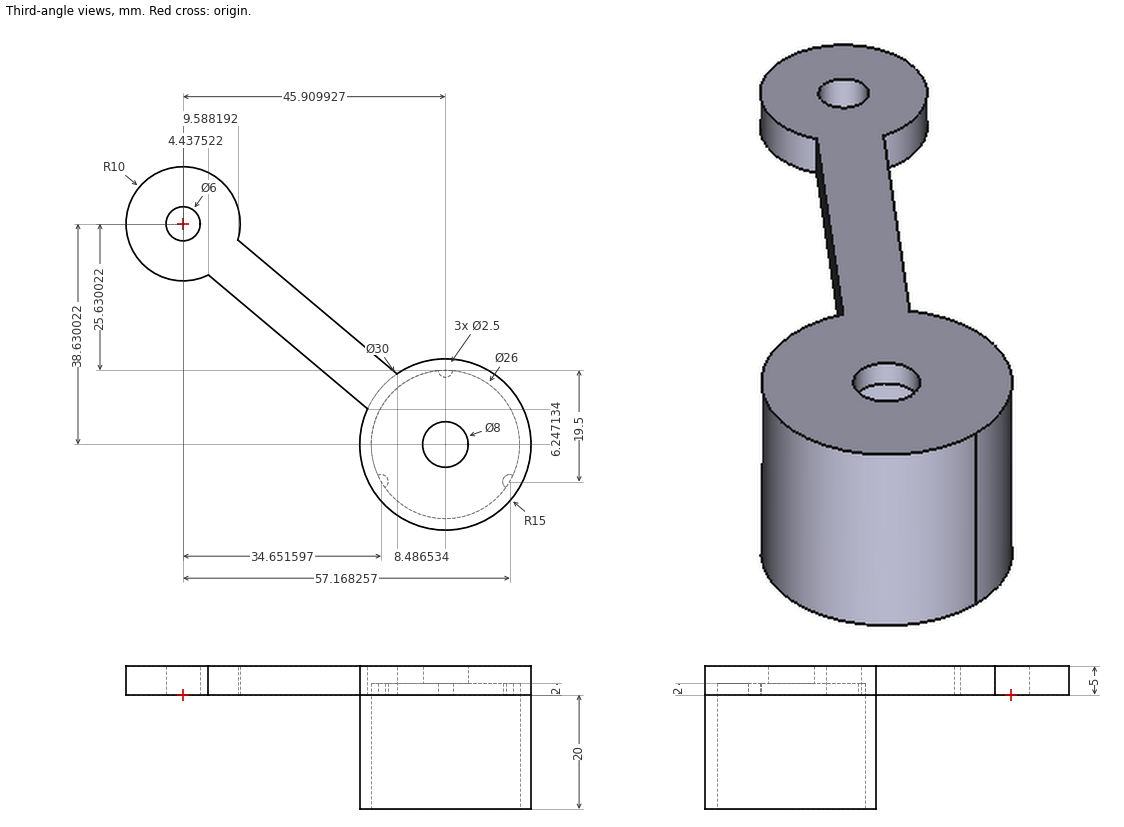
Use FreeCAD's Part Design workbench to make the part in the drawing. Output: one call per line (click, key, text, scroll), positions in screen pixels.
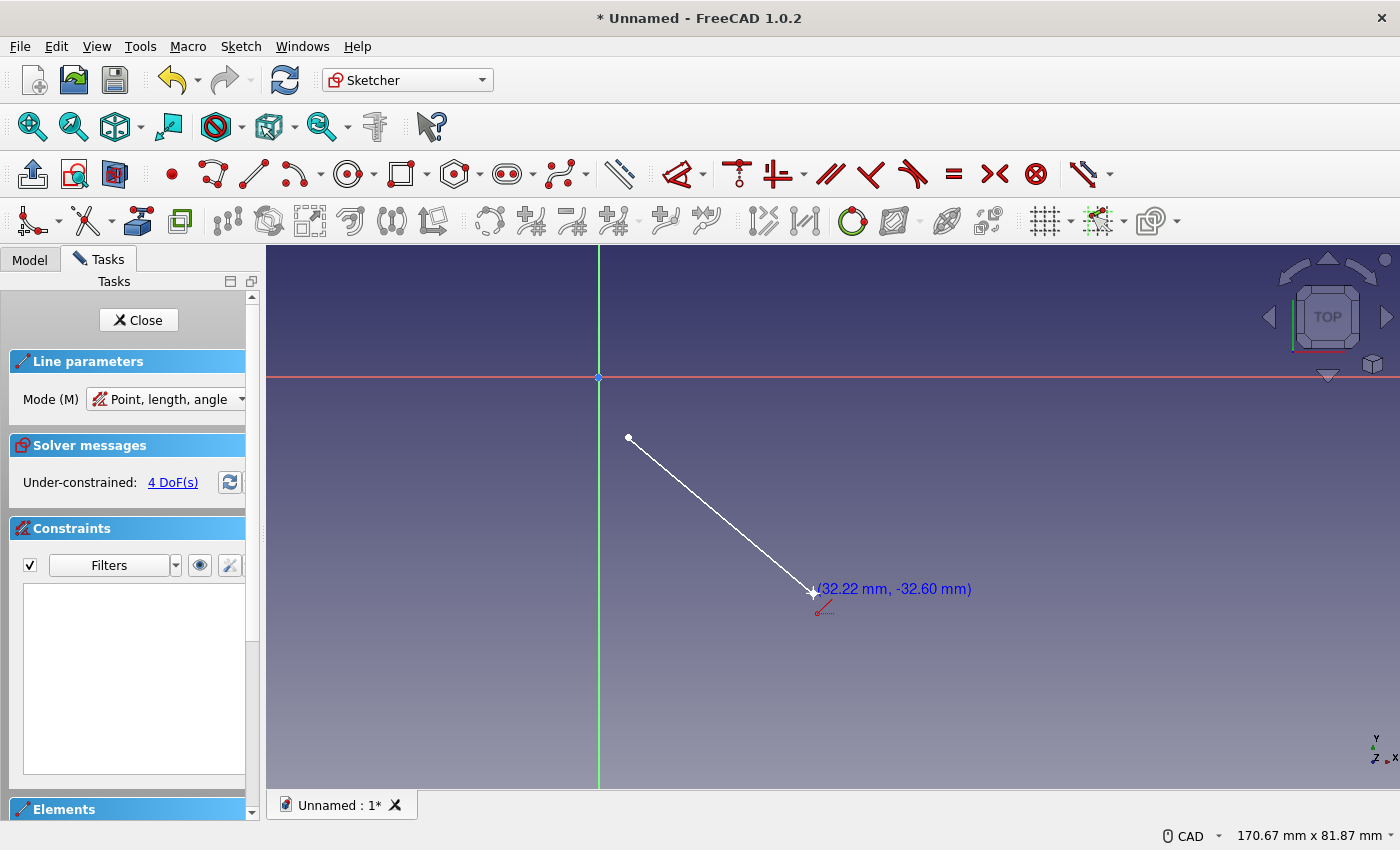
click(848, 552)
click(663, 396)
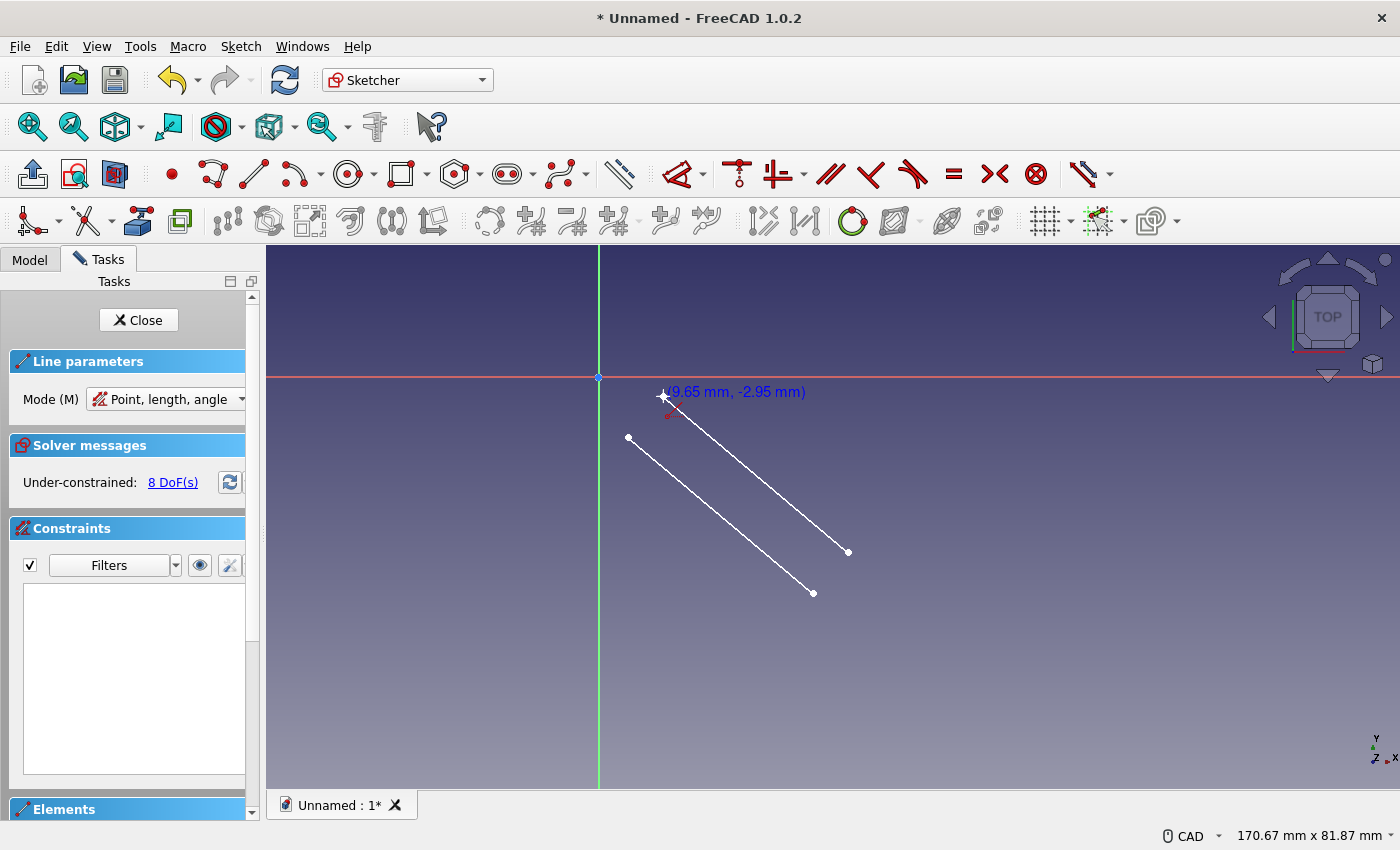
key(g)
key(3)
key(a)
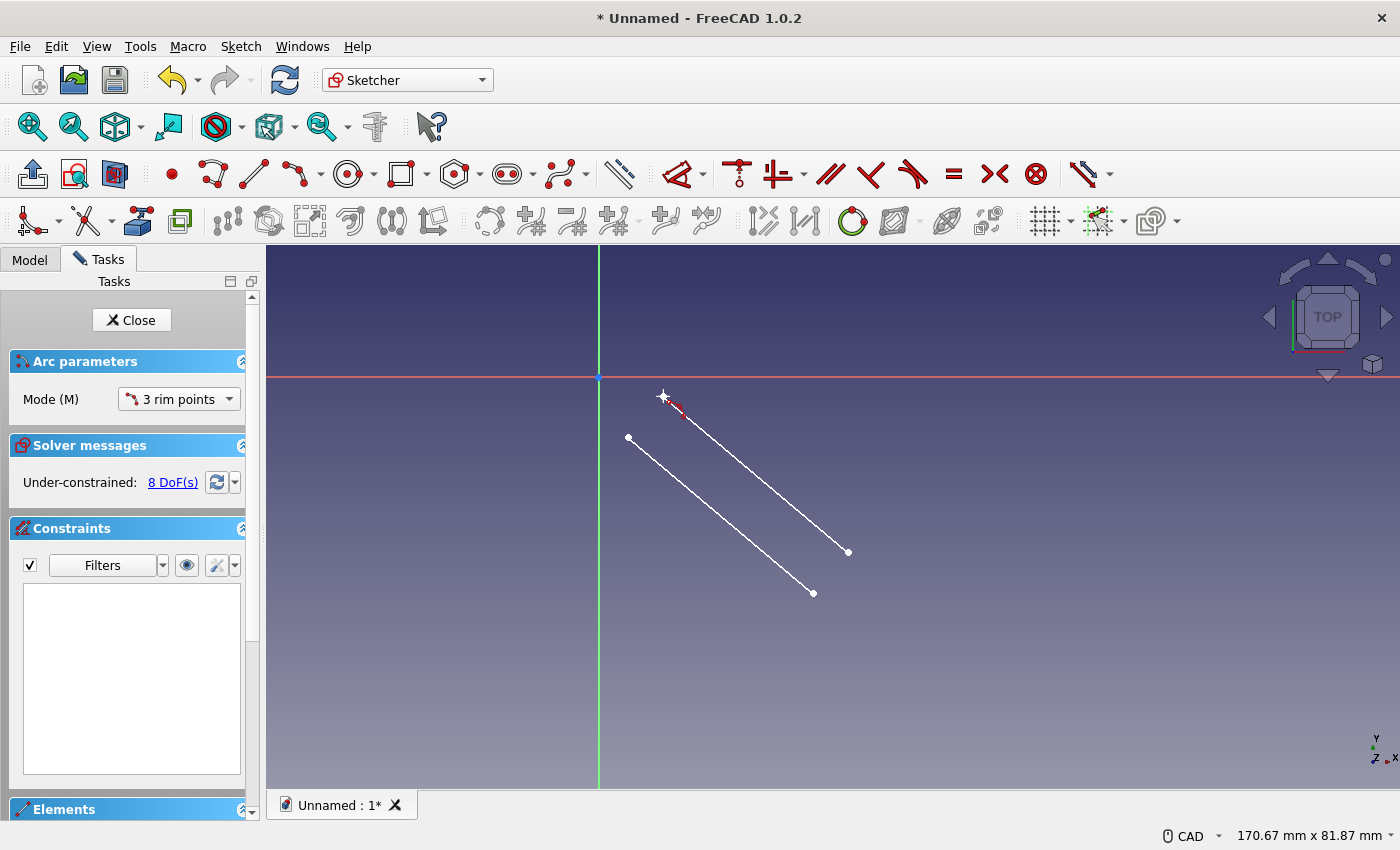
click(813, 594)
click(848, 553)
click(980, 698)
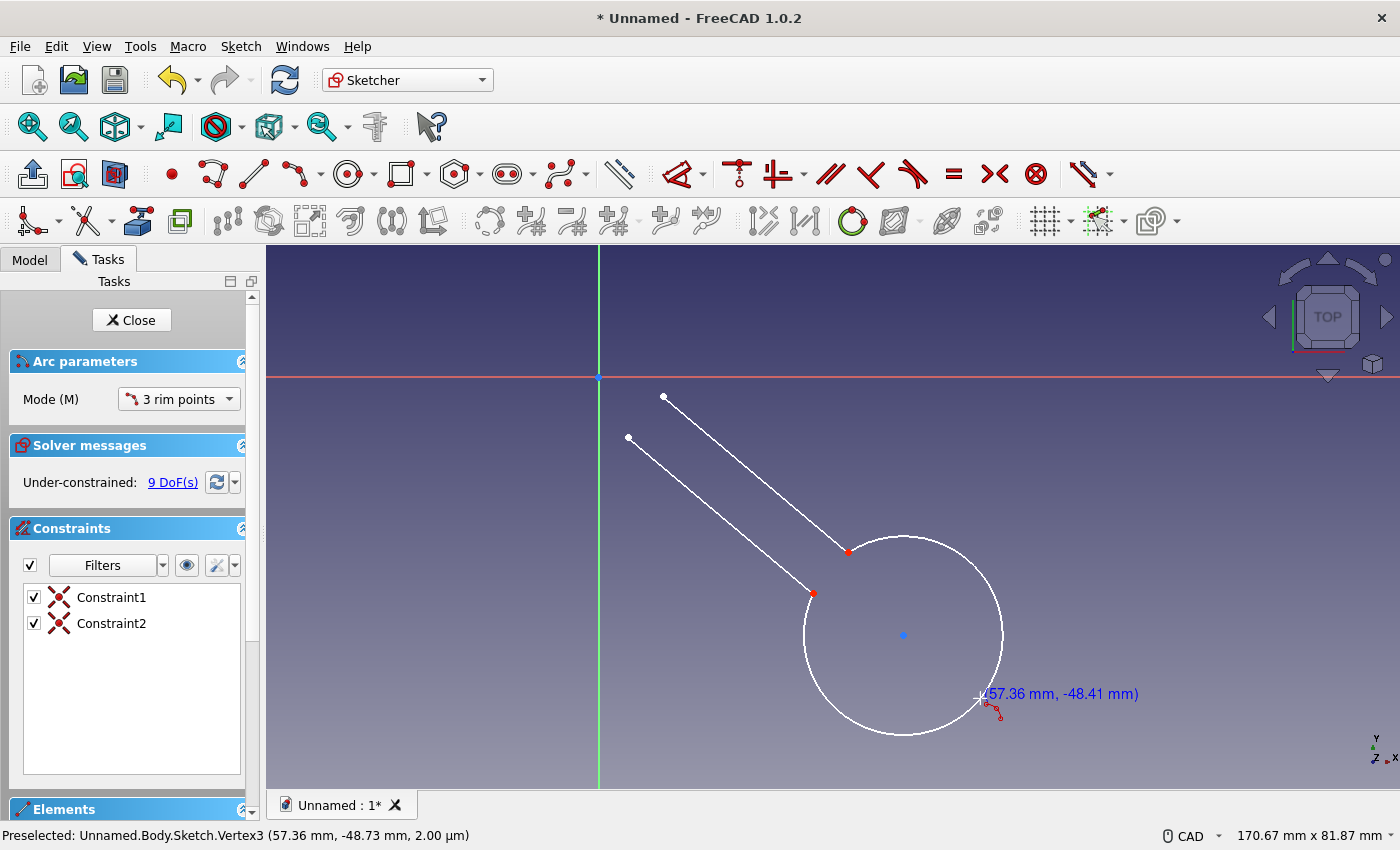
click(663, 397)
click(628, 438)
click(548, 335)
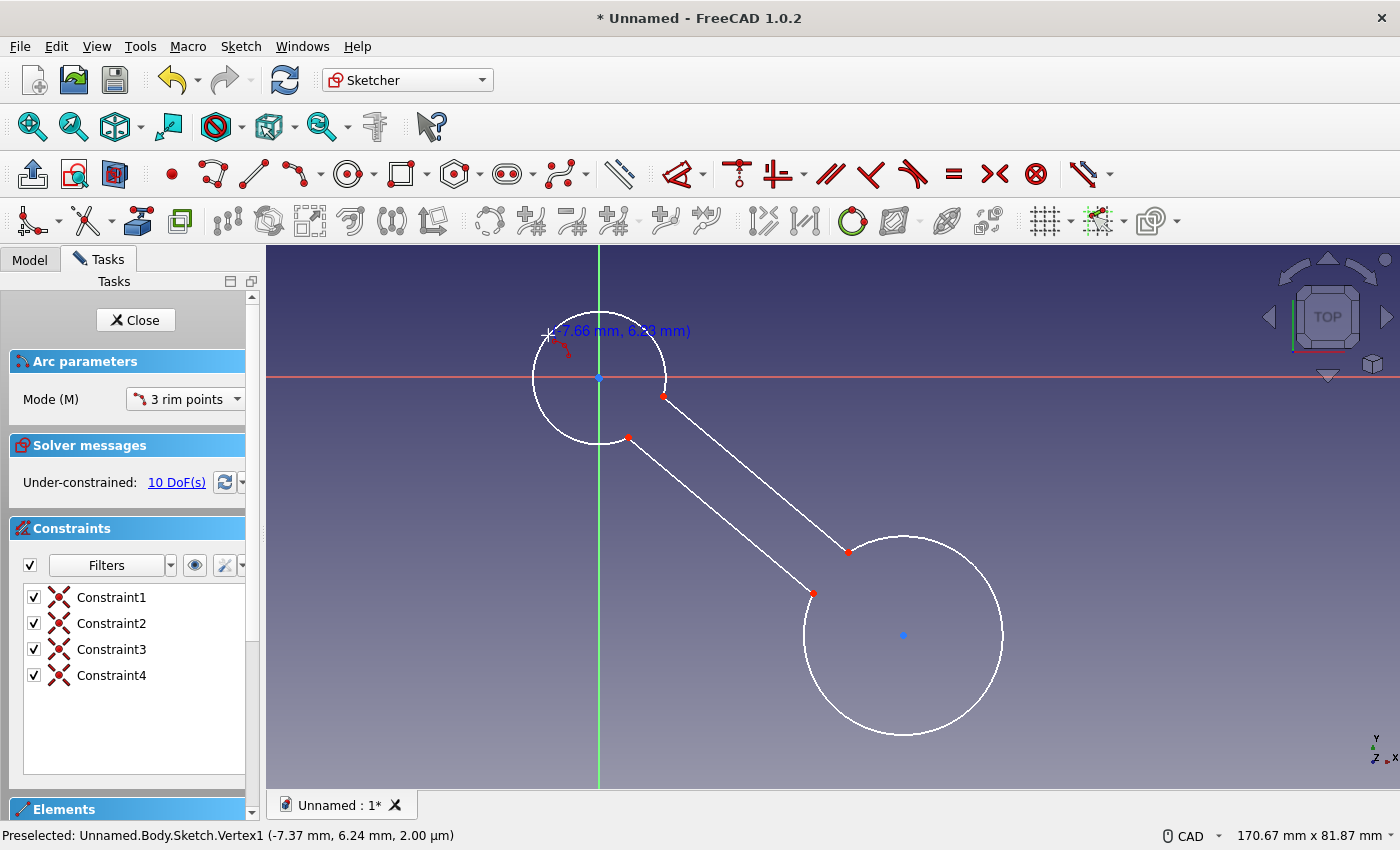
click(348, 174)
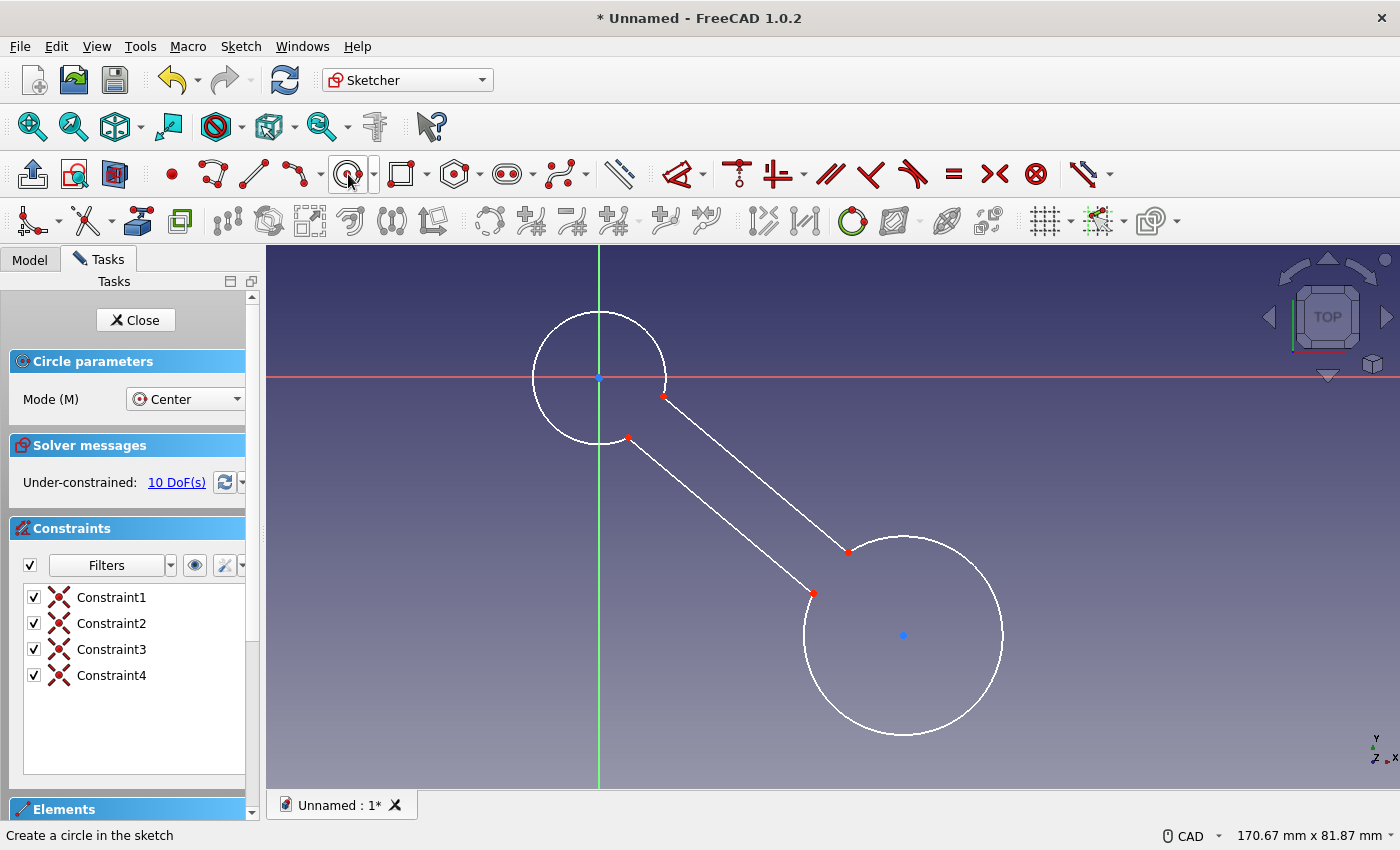
click(904, 634)
move(923, 615)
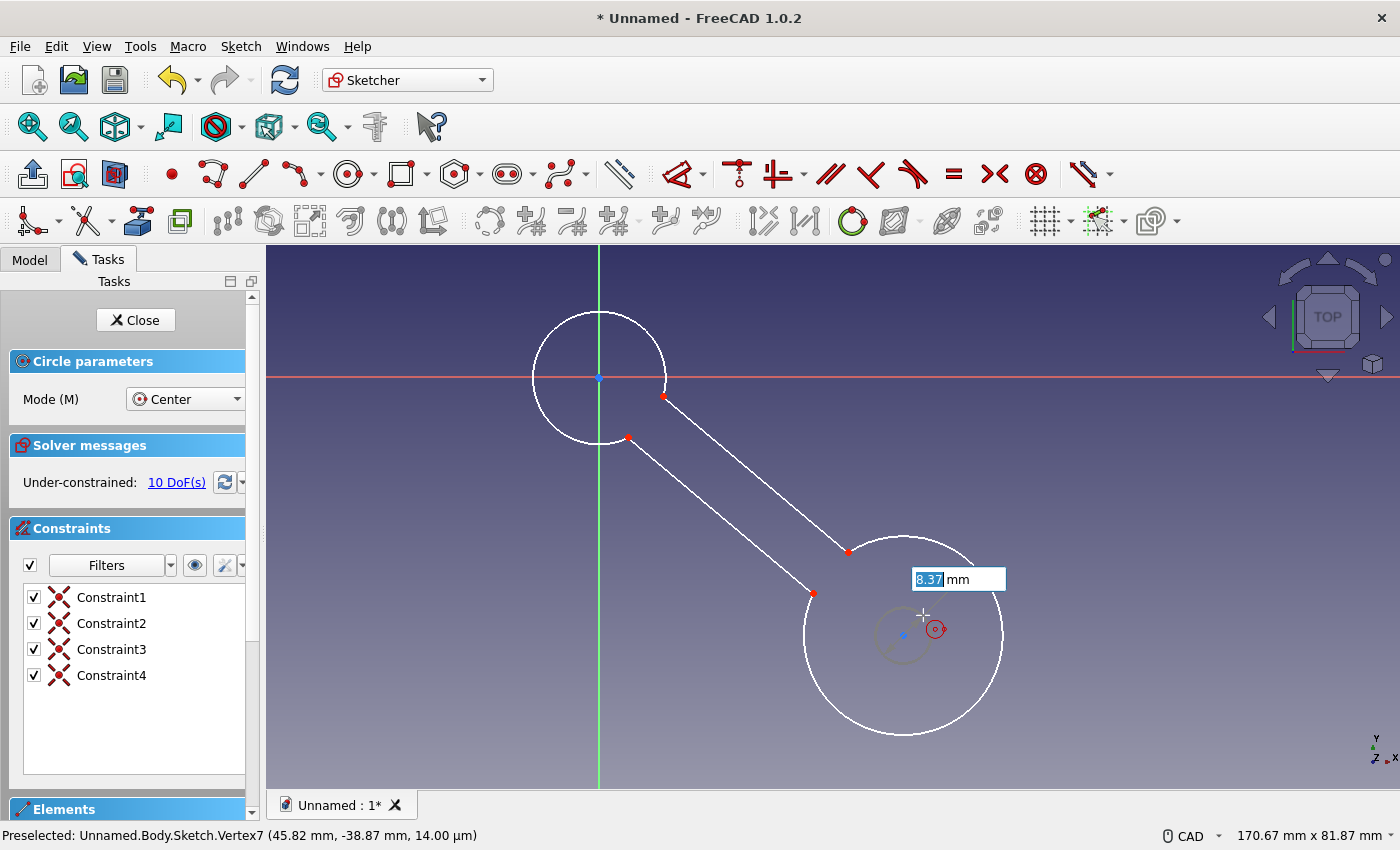
text(8)
key(Return)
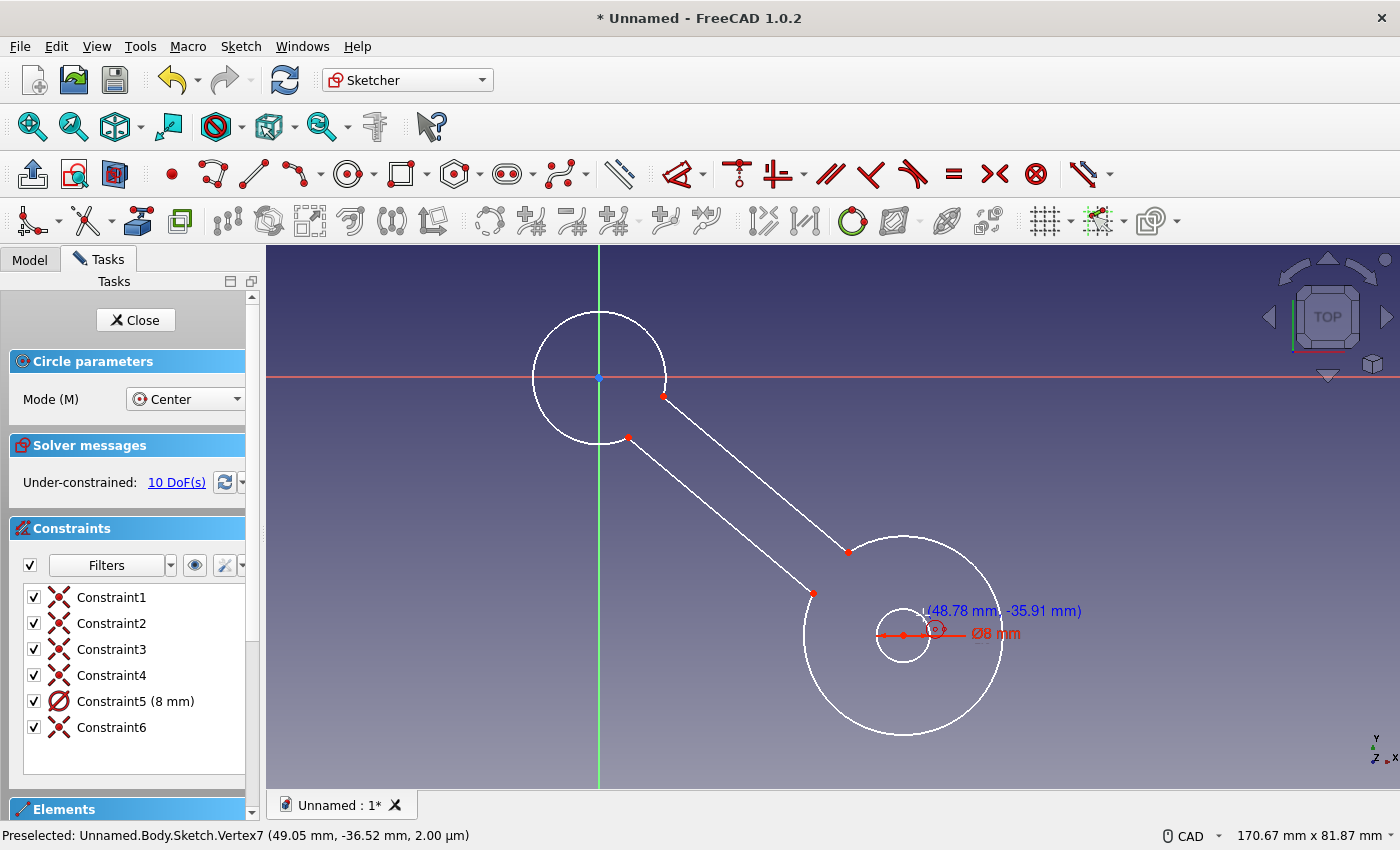
click(599, 377)
move(613, 363)